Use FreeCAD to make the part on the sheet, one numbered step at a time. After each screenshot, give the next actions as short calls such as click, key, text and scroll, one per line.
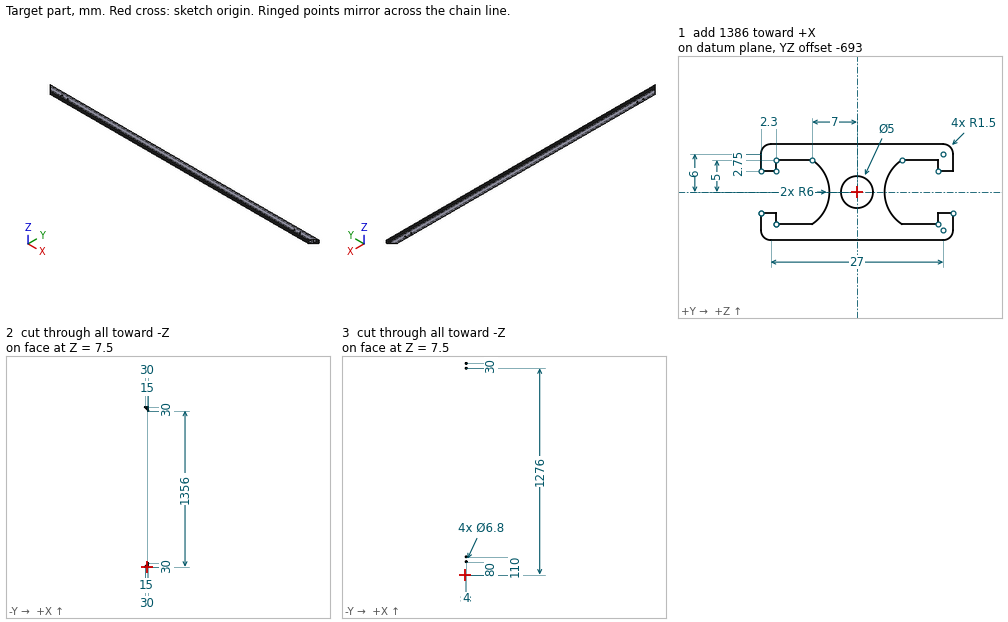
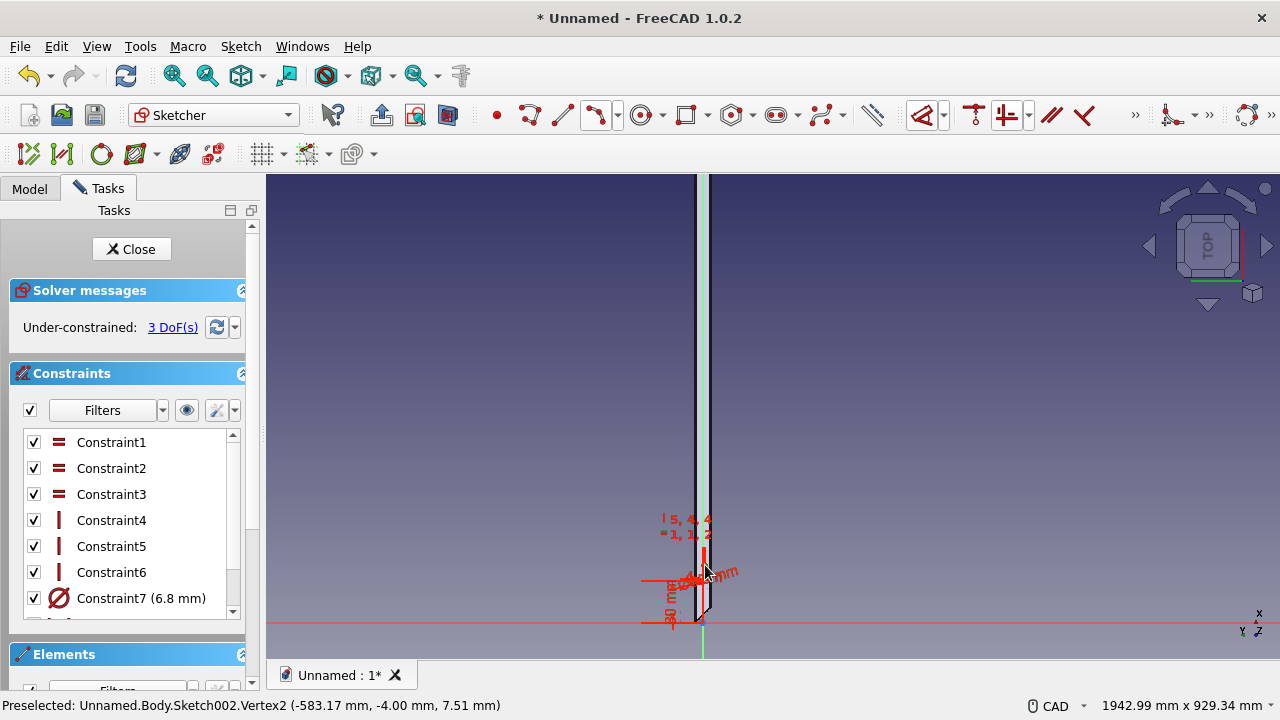
key(i)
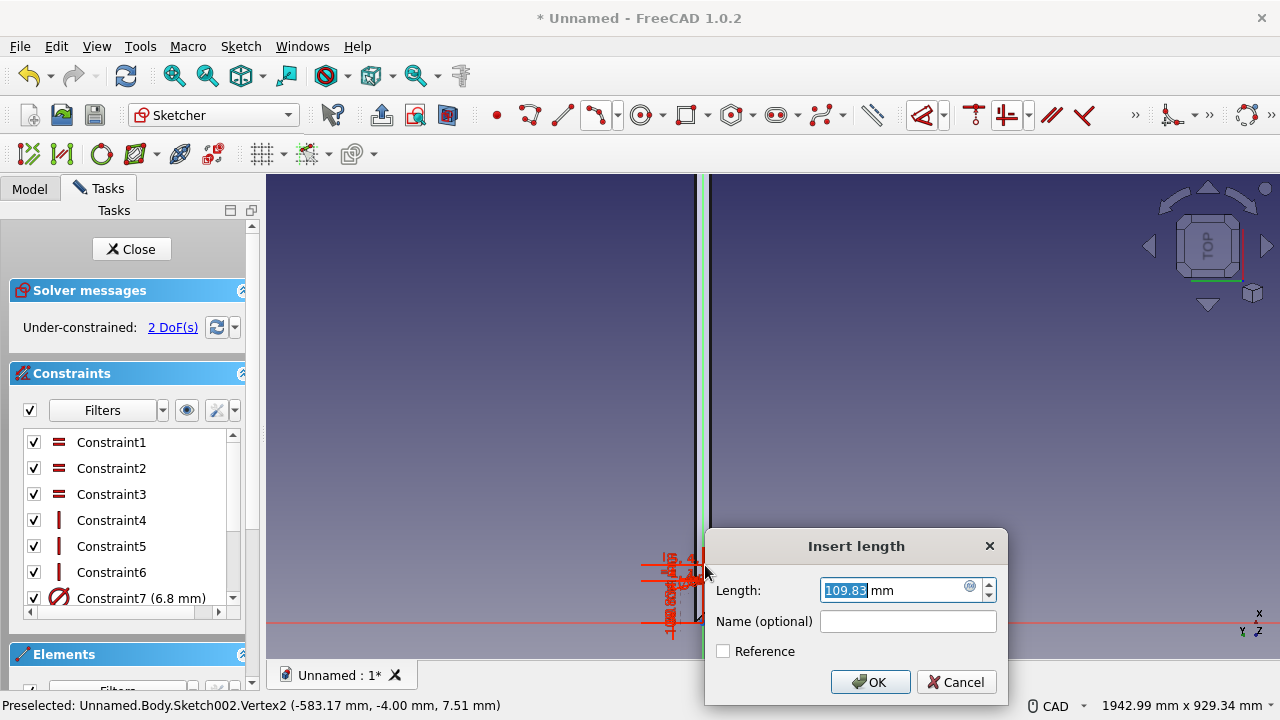
text(110)
key(Return)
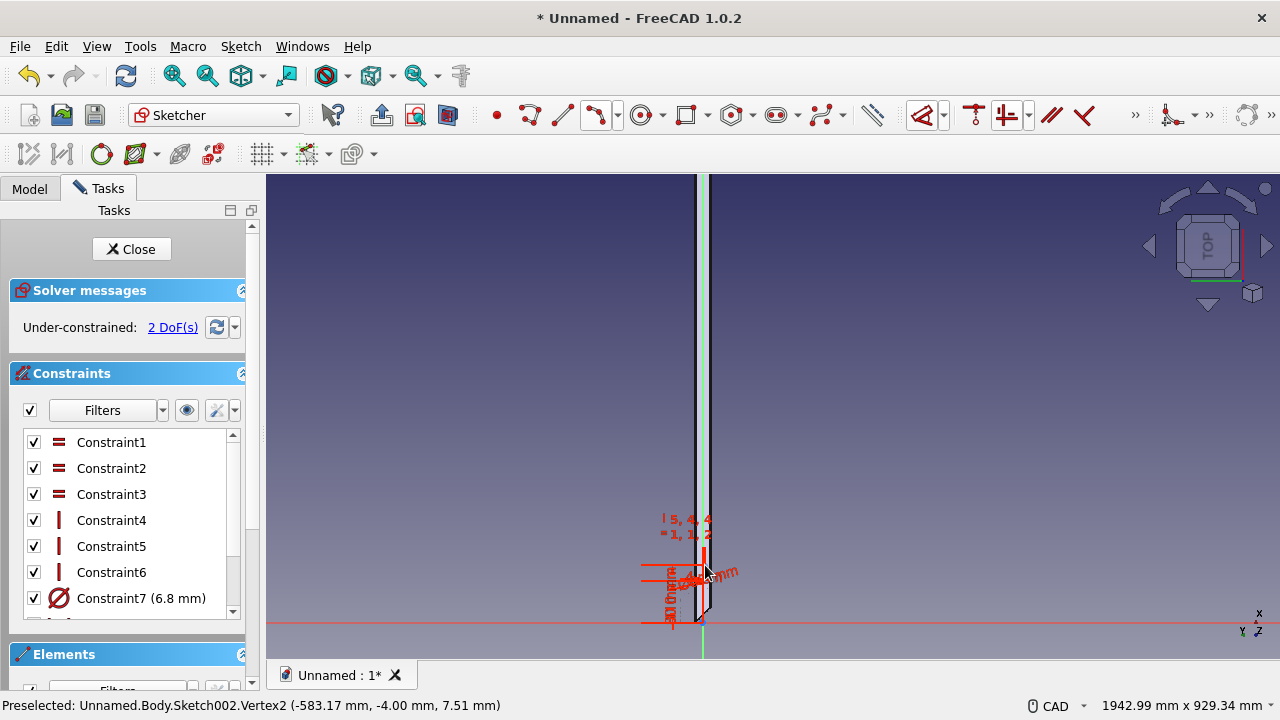
scroll(704, 527, down, 4)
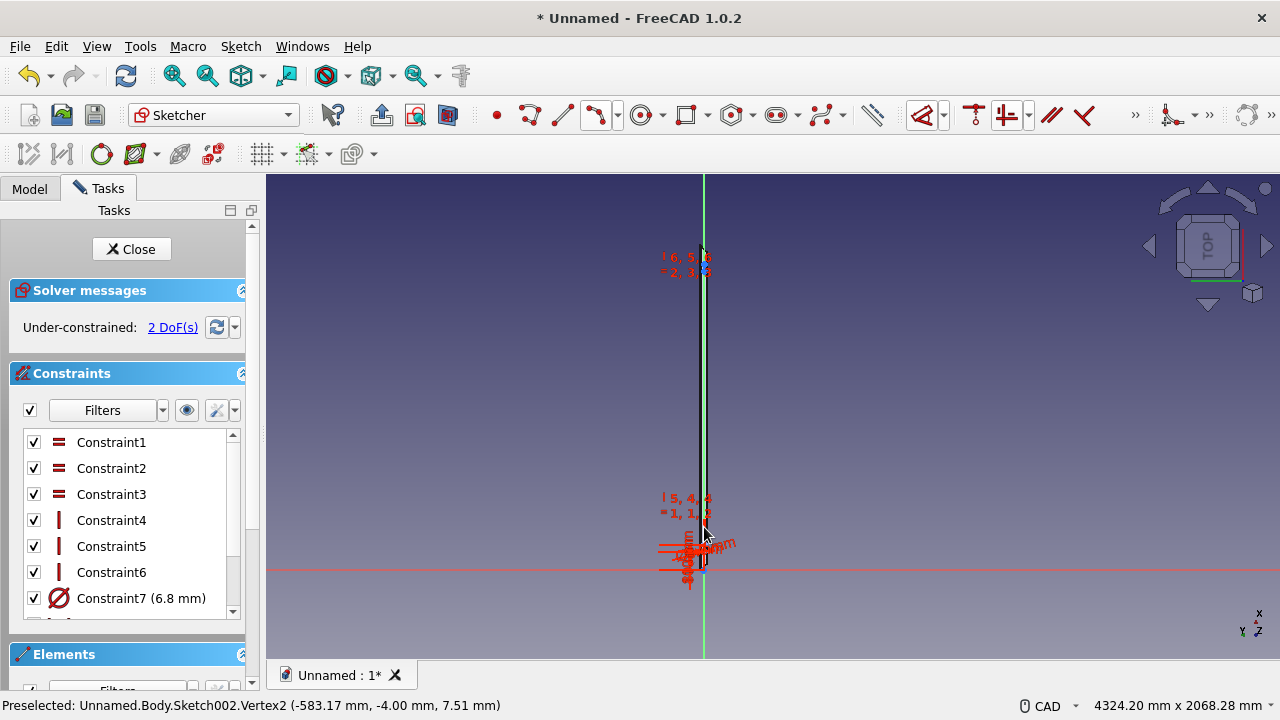
scroll(705, 271, up, 9)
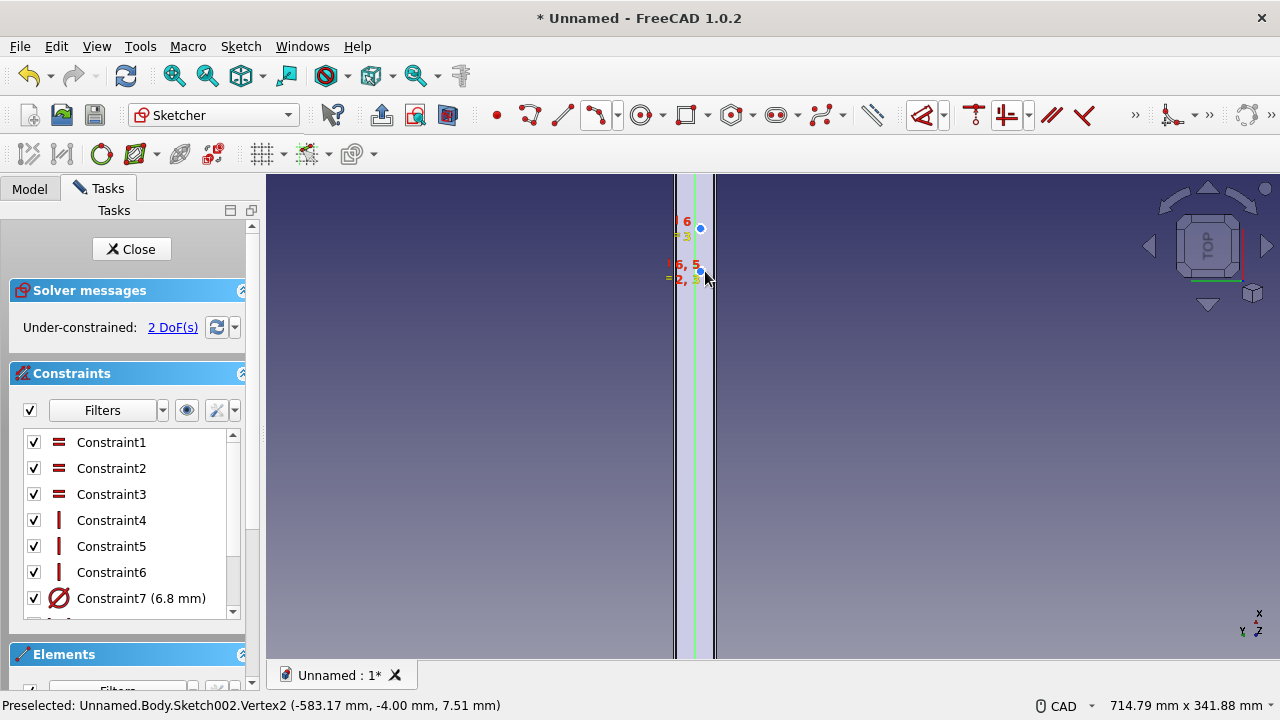
click(701, 271)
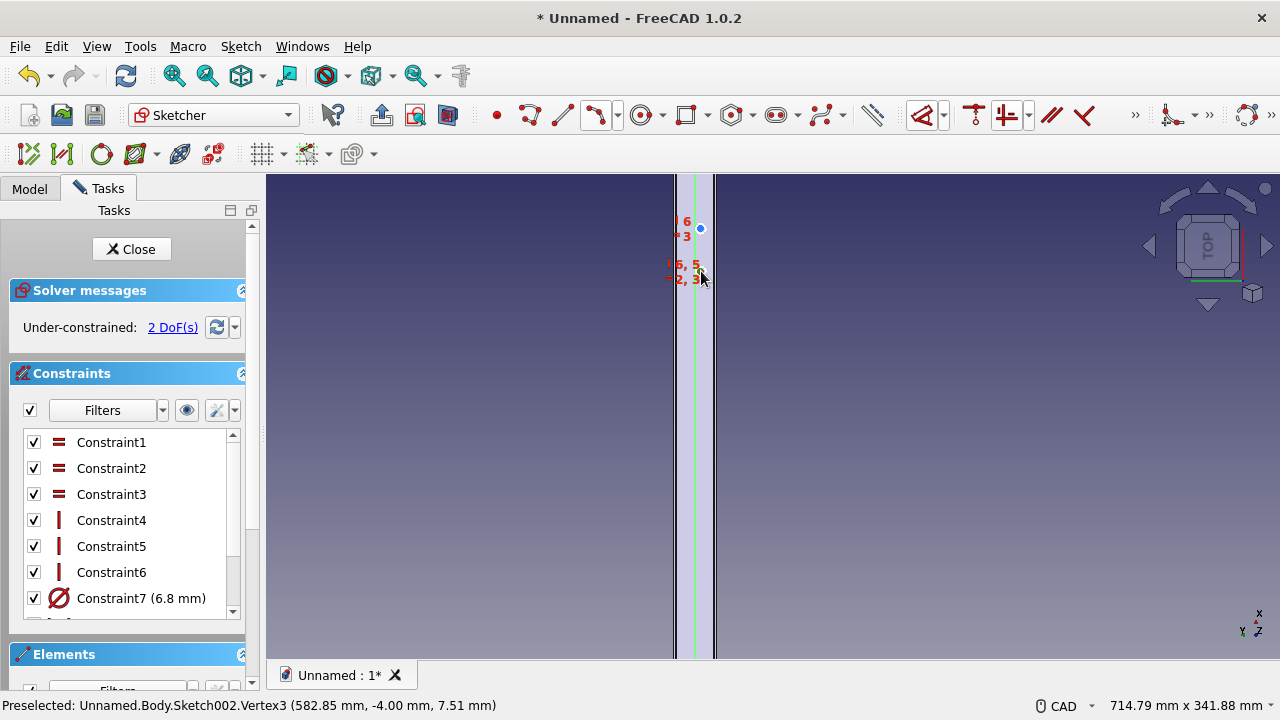
click(701, 229)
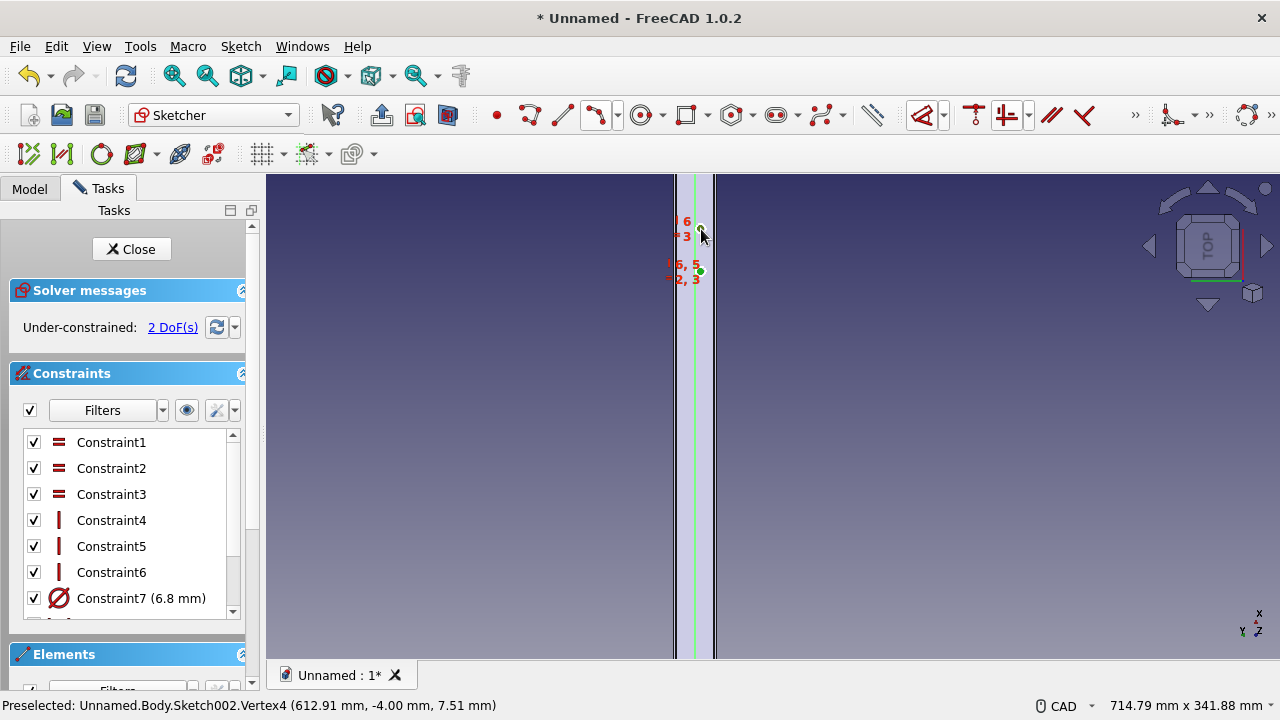
click(944, 116)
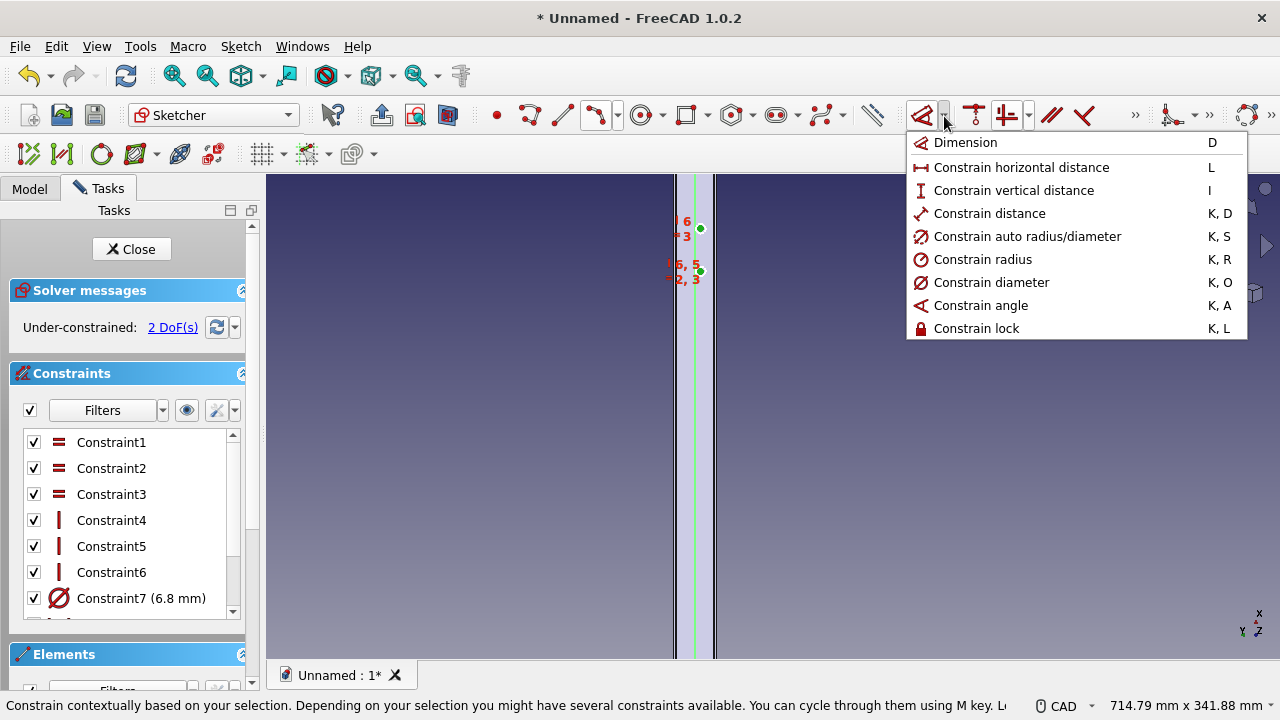
click(1077, 190)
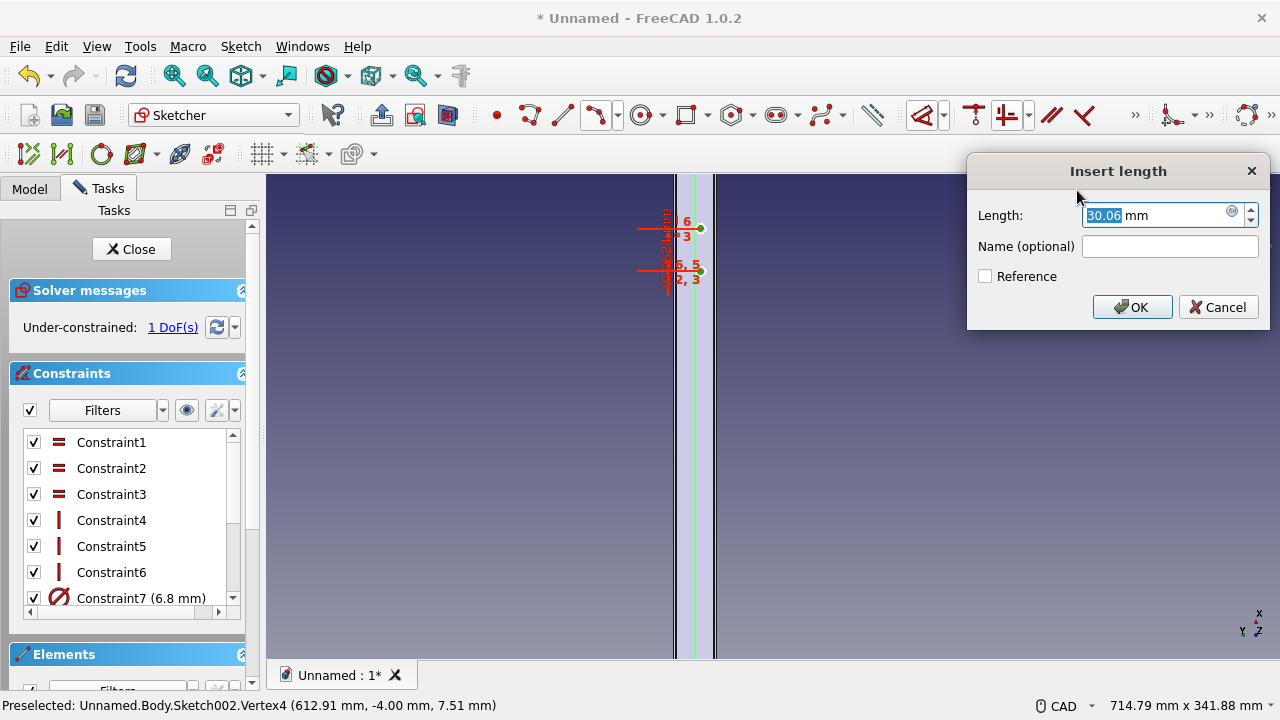
text(30)
key(Return)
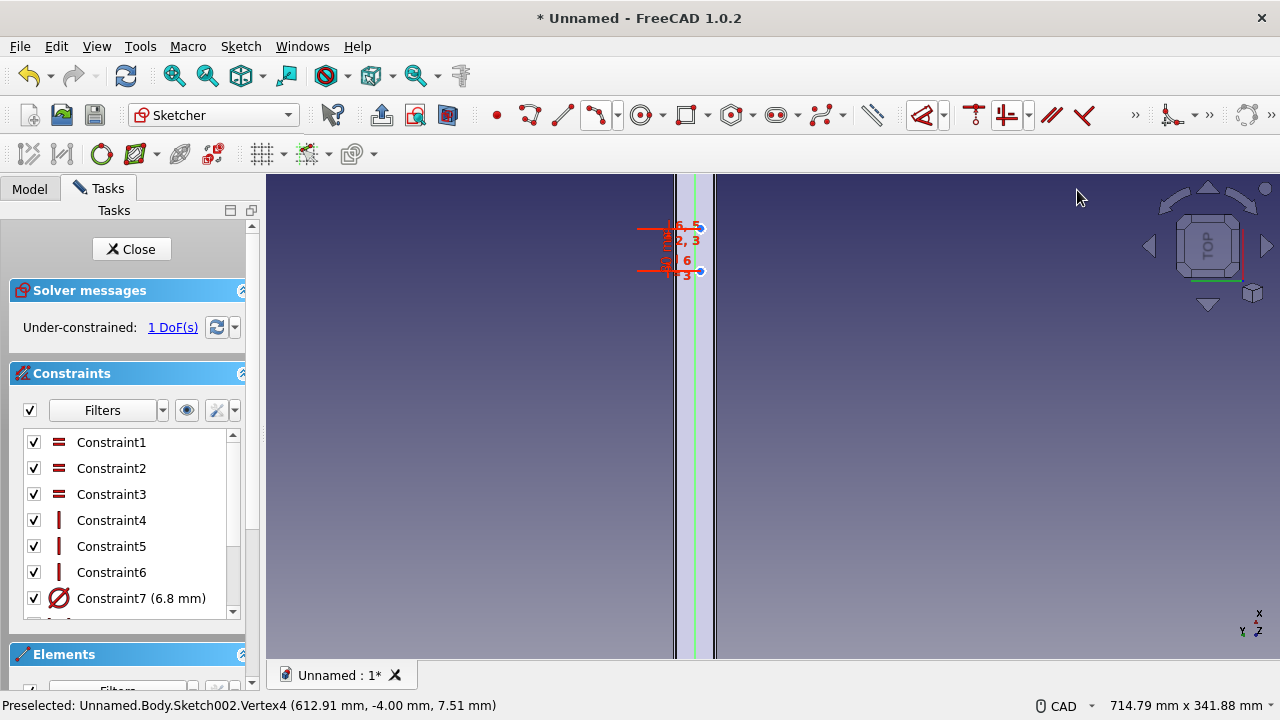
scroll(705, 271, down, 9)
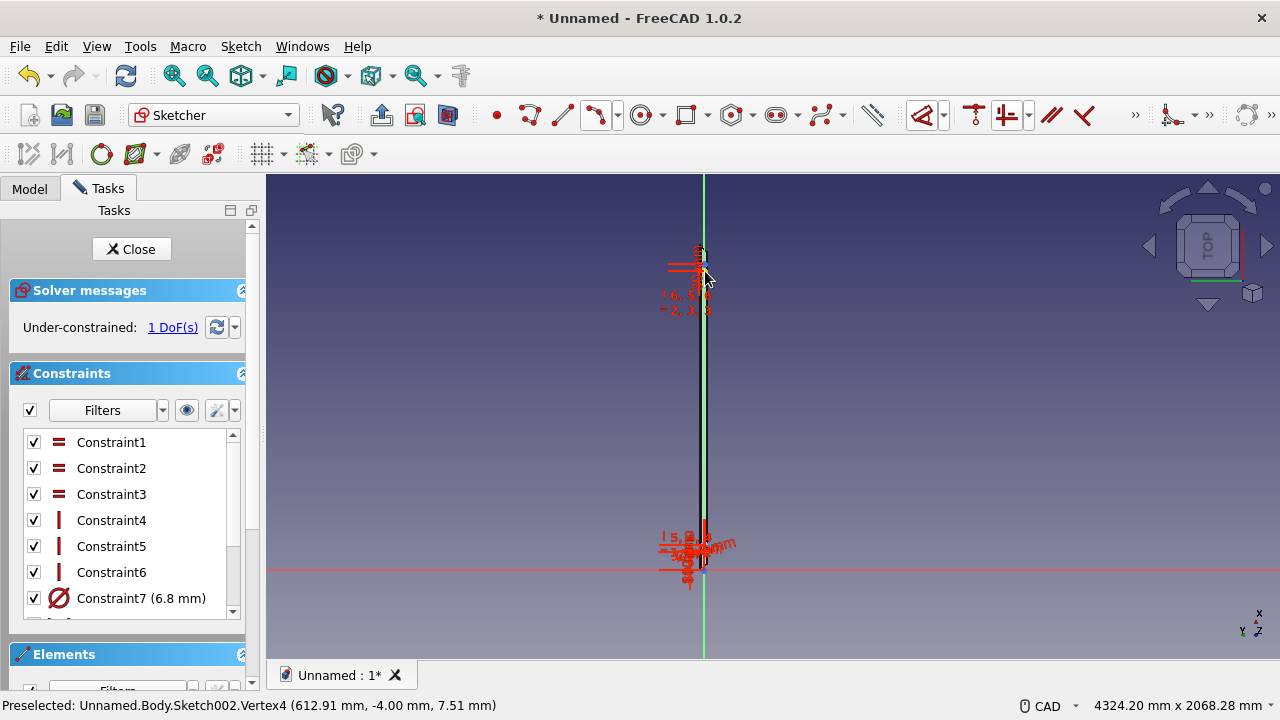
scroll(705, 271, up, 3)